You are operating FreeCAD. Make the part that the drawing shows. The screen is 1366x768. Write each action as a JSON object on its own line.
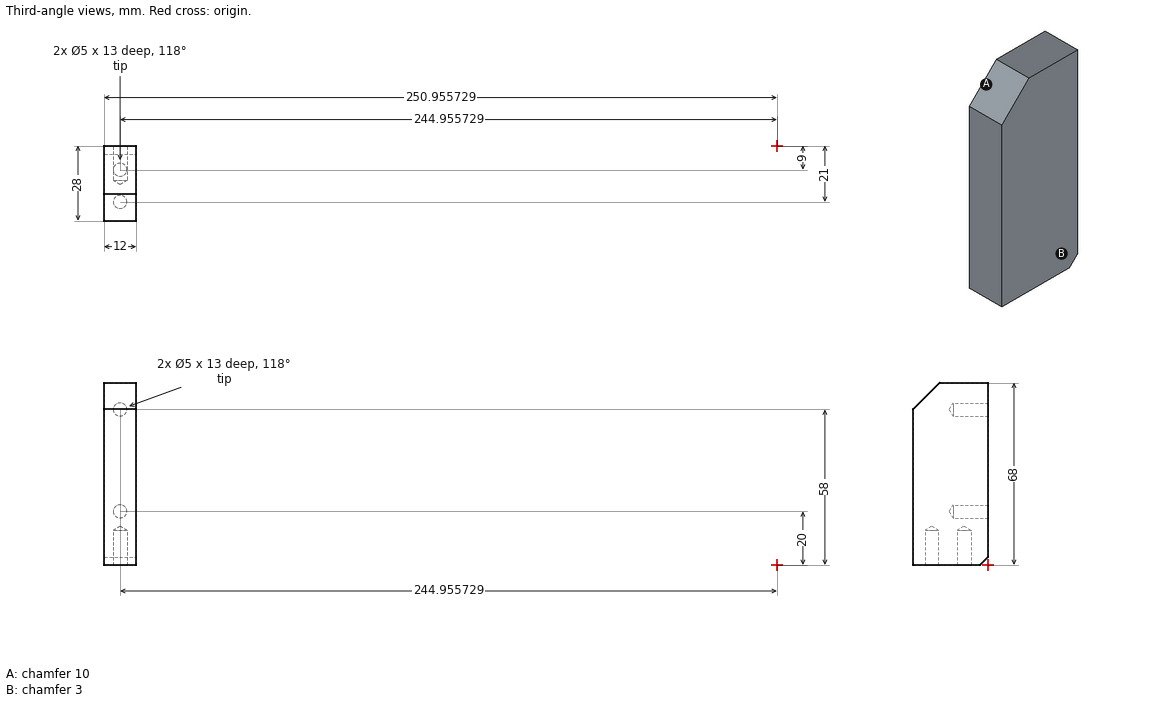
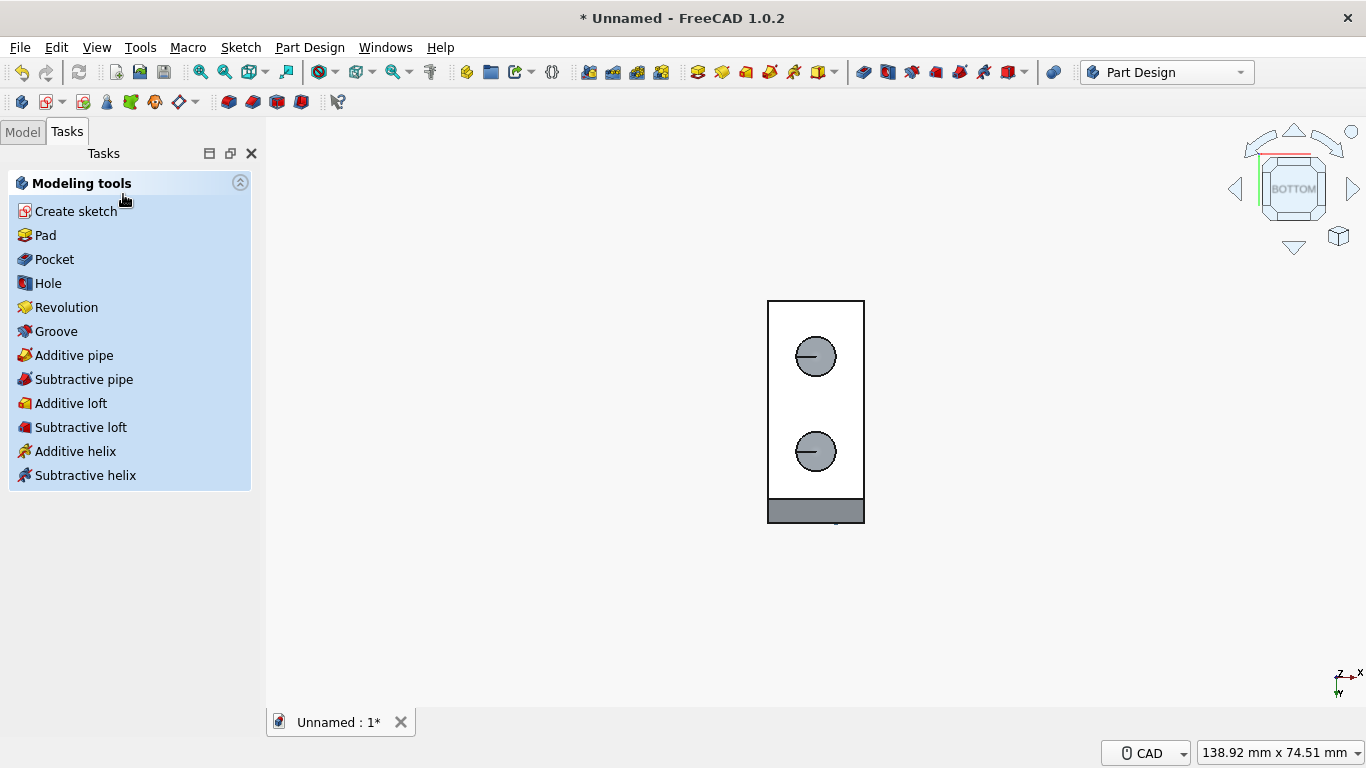
{"action": "left_click", "coordinate": [888, 72]}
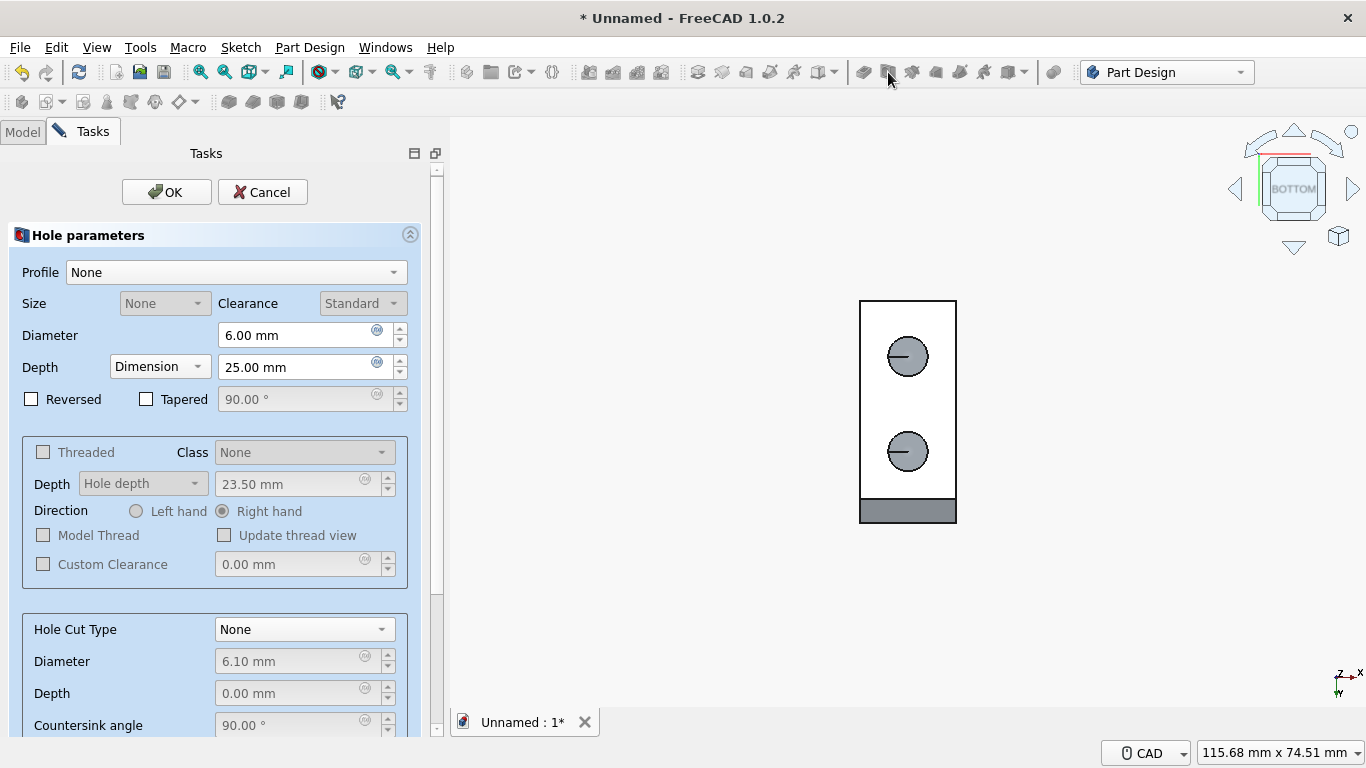
{"action": "triple_click", "coordinate": [305, 335]}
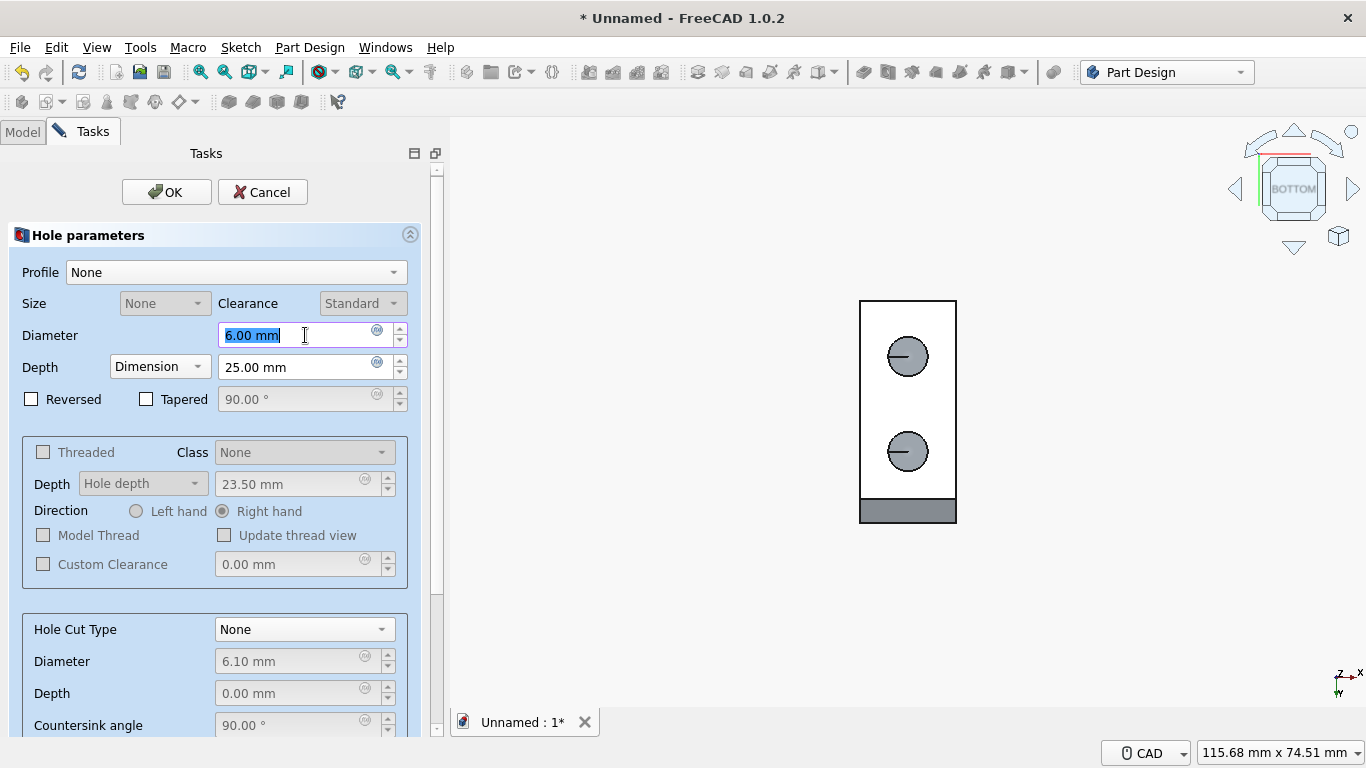
{"action": "type", "text": "5"}
{"action": "key", "text": "Tab"}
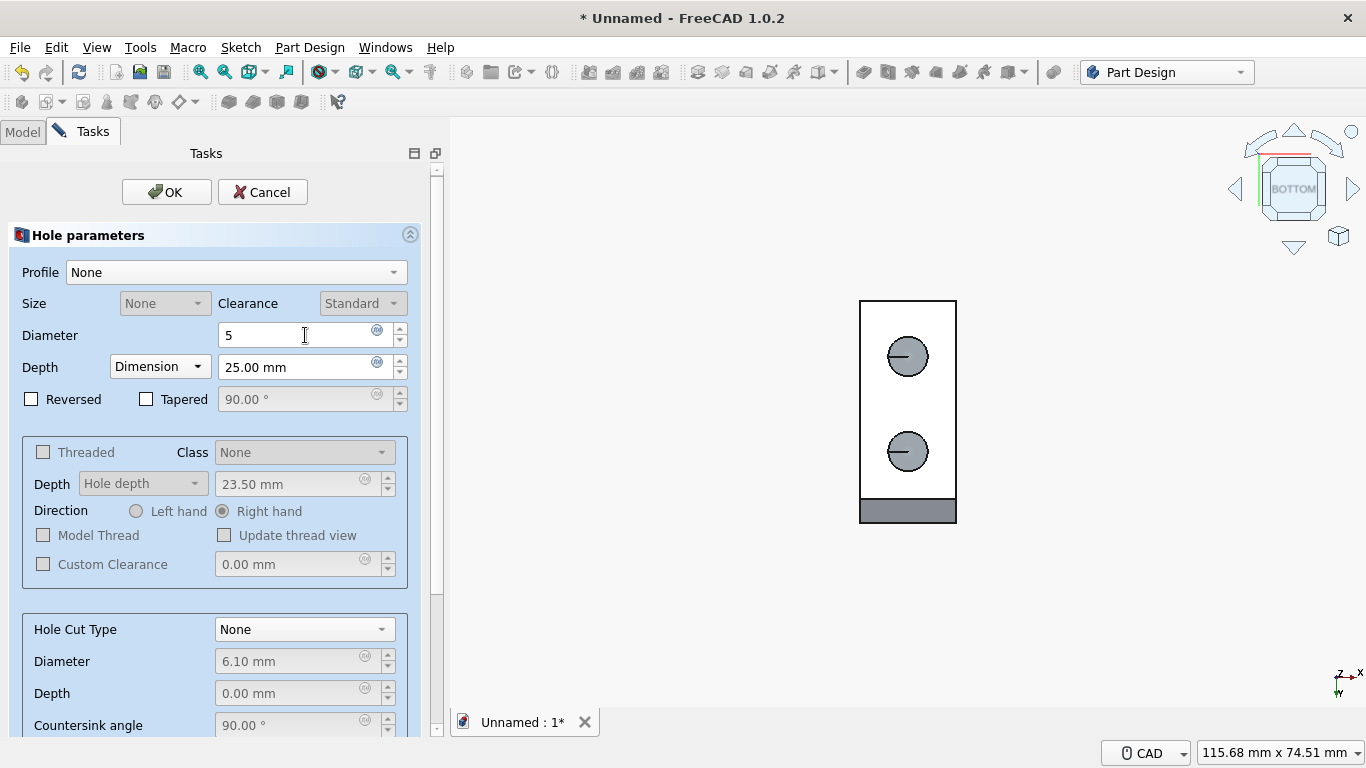
{"action": "triple_click", "coordinate": [305, 367]}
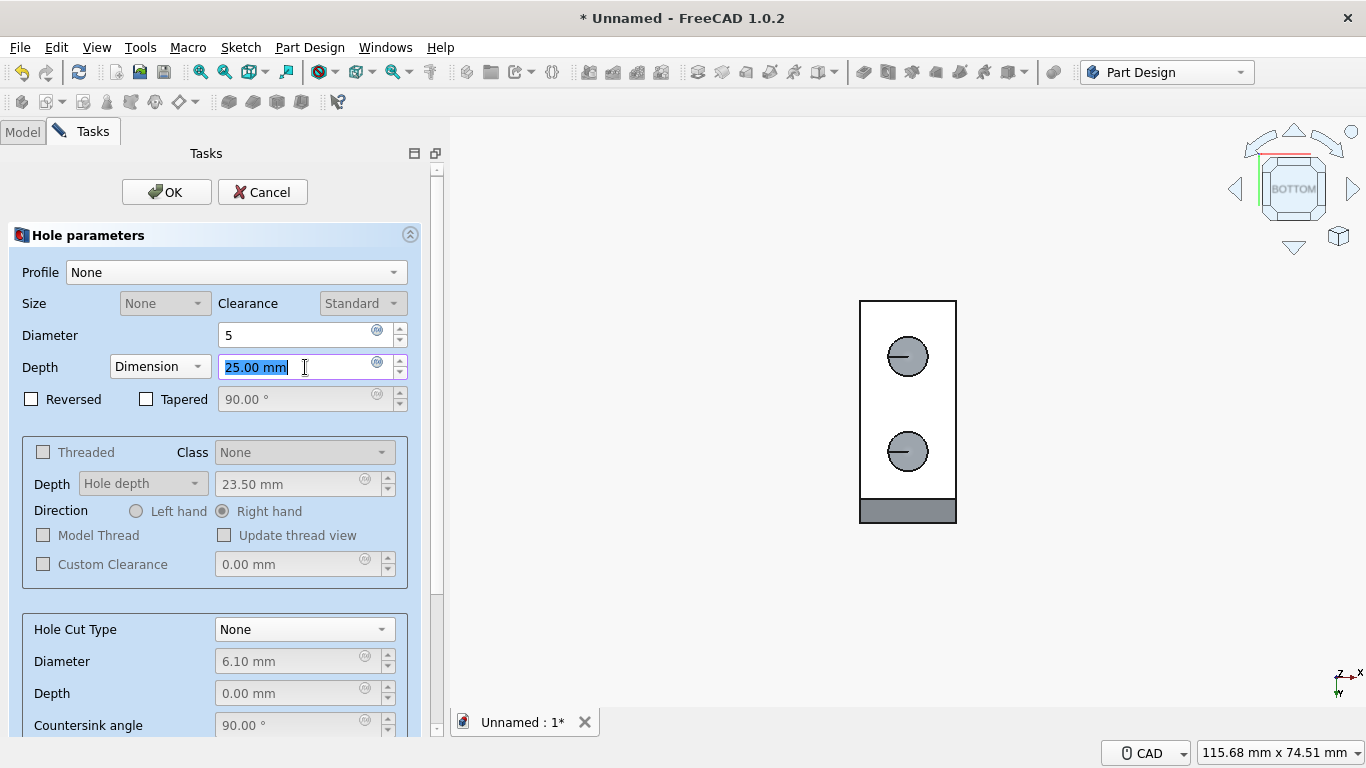
{"action": "type", "text": "13"}
{"action": "key", "text": "Tab"}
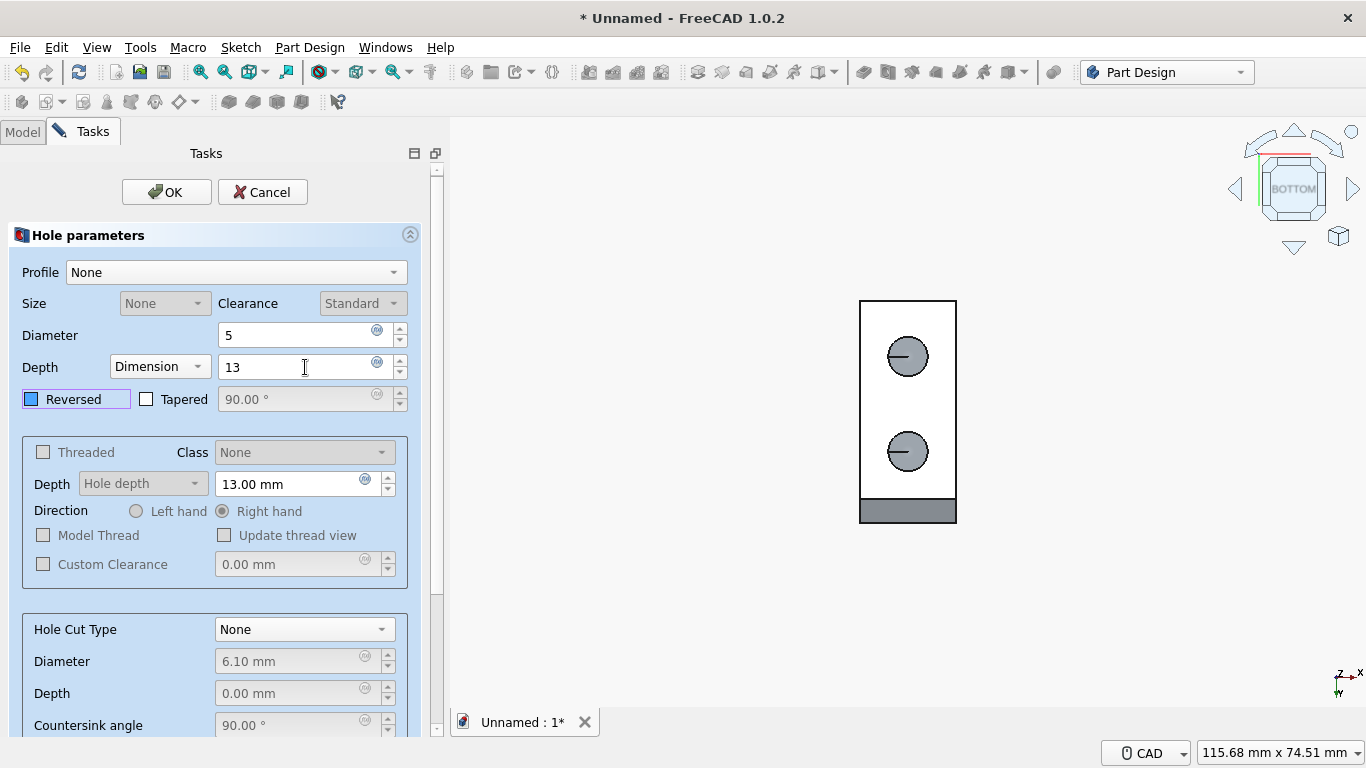
{"action": "left_click", "coordinate": [30, 399]}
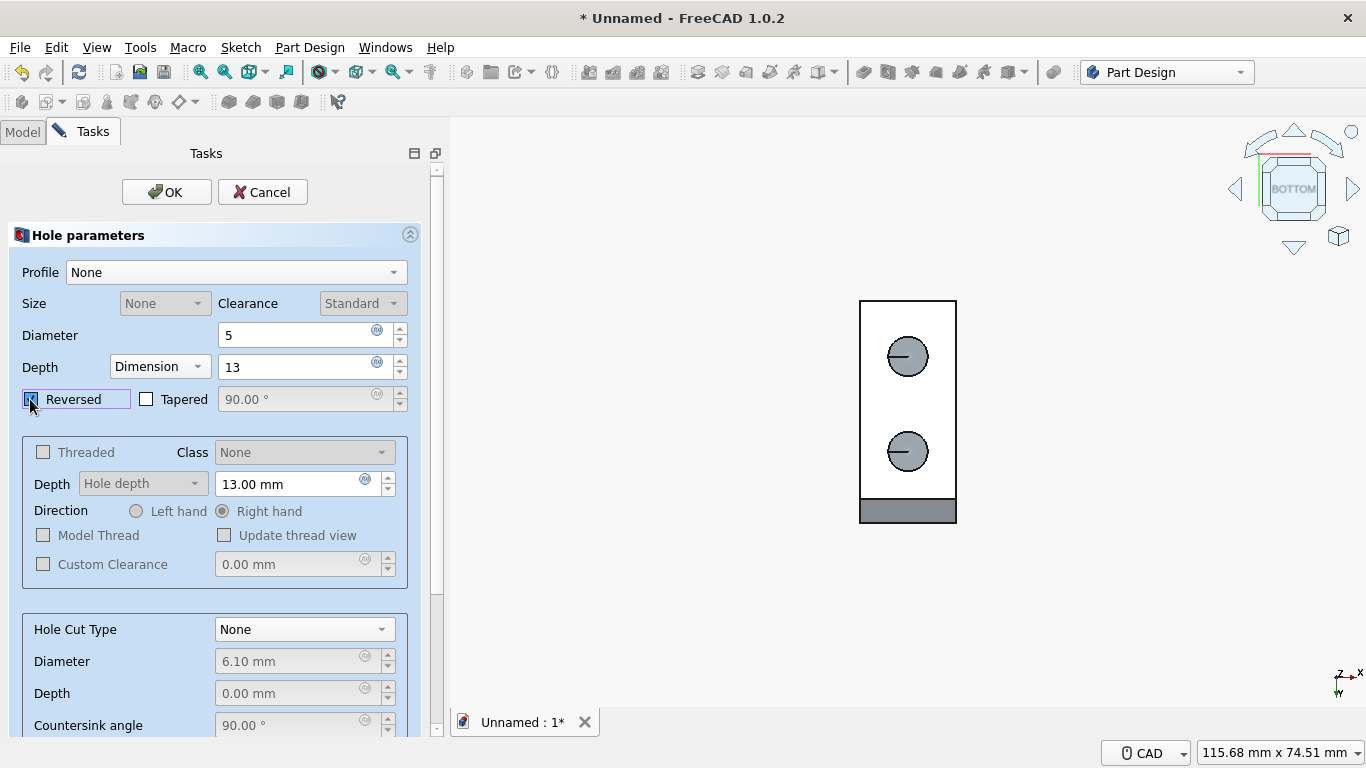
{"action": "left_click", "coordinate": [167, 192]}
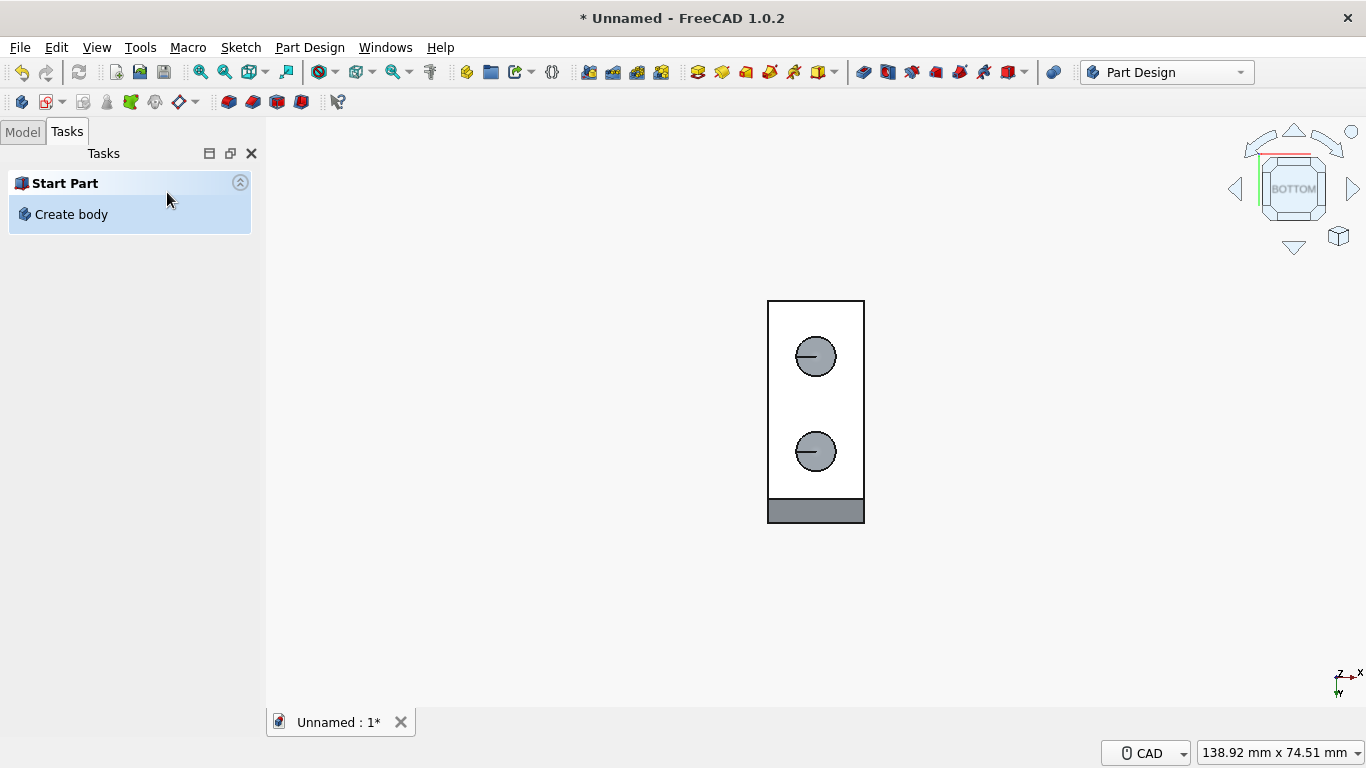
{"action": "key", "text": "0"}